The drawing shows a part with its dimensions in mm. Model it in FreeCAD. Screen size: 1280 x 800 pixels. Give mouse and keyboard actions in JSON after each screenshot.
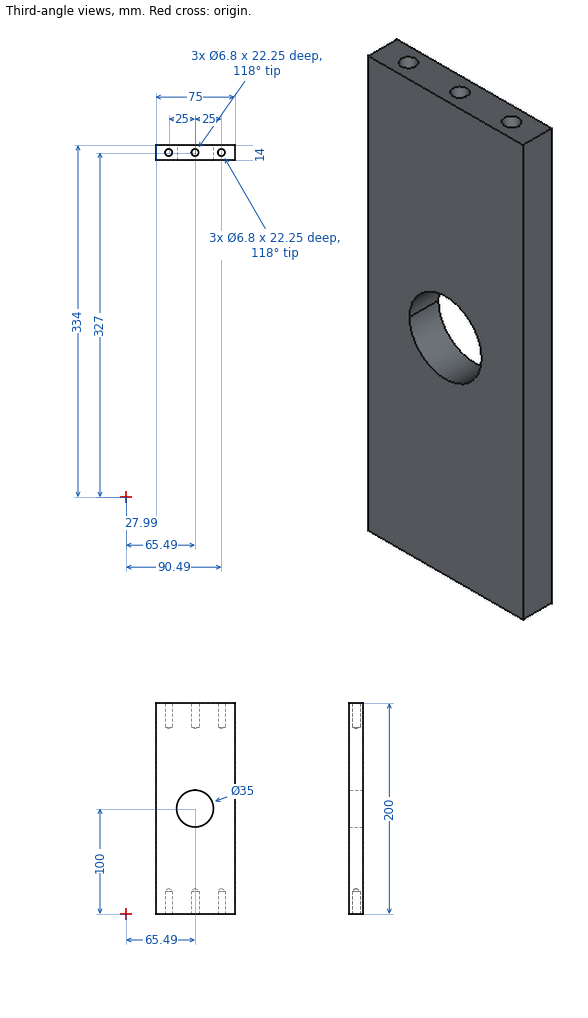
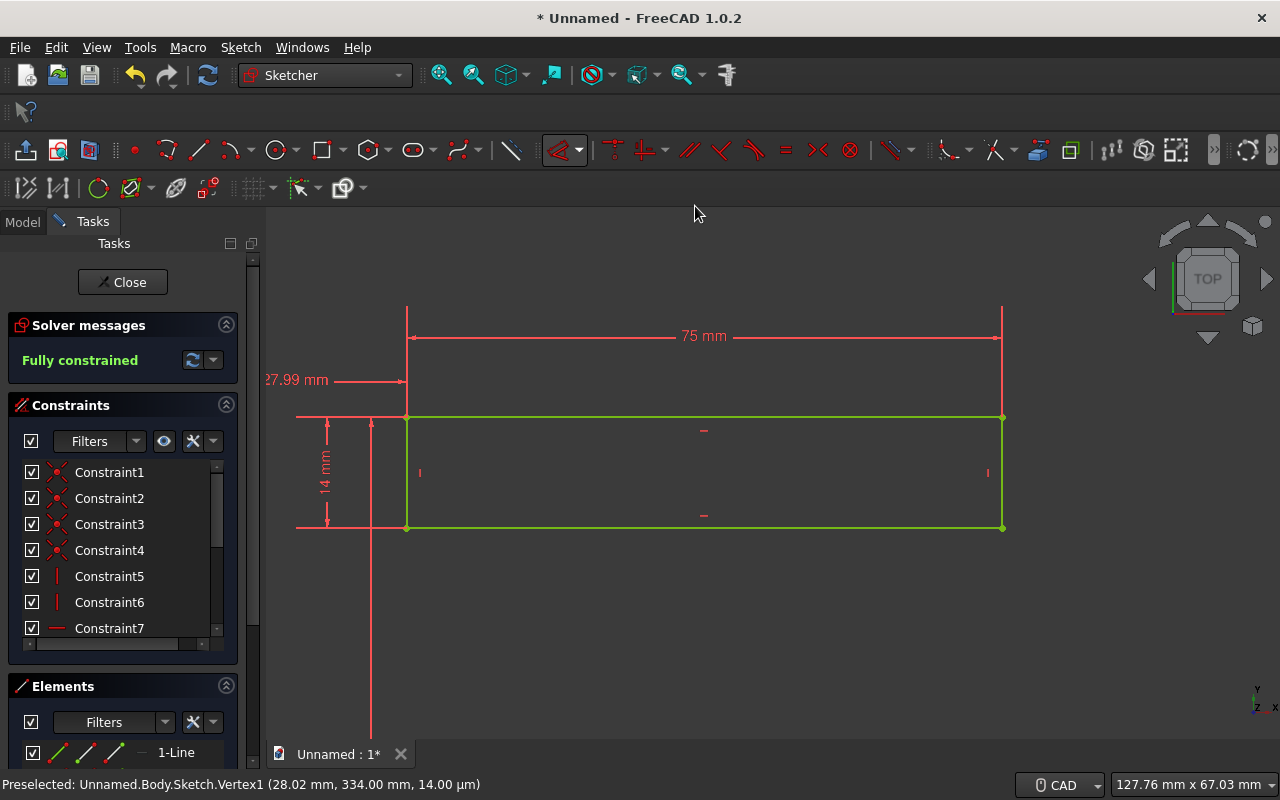
{"action": "left_click", "coordinate": [123, 282]}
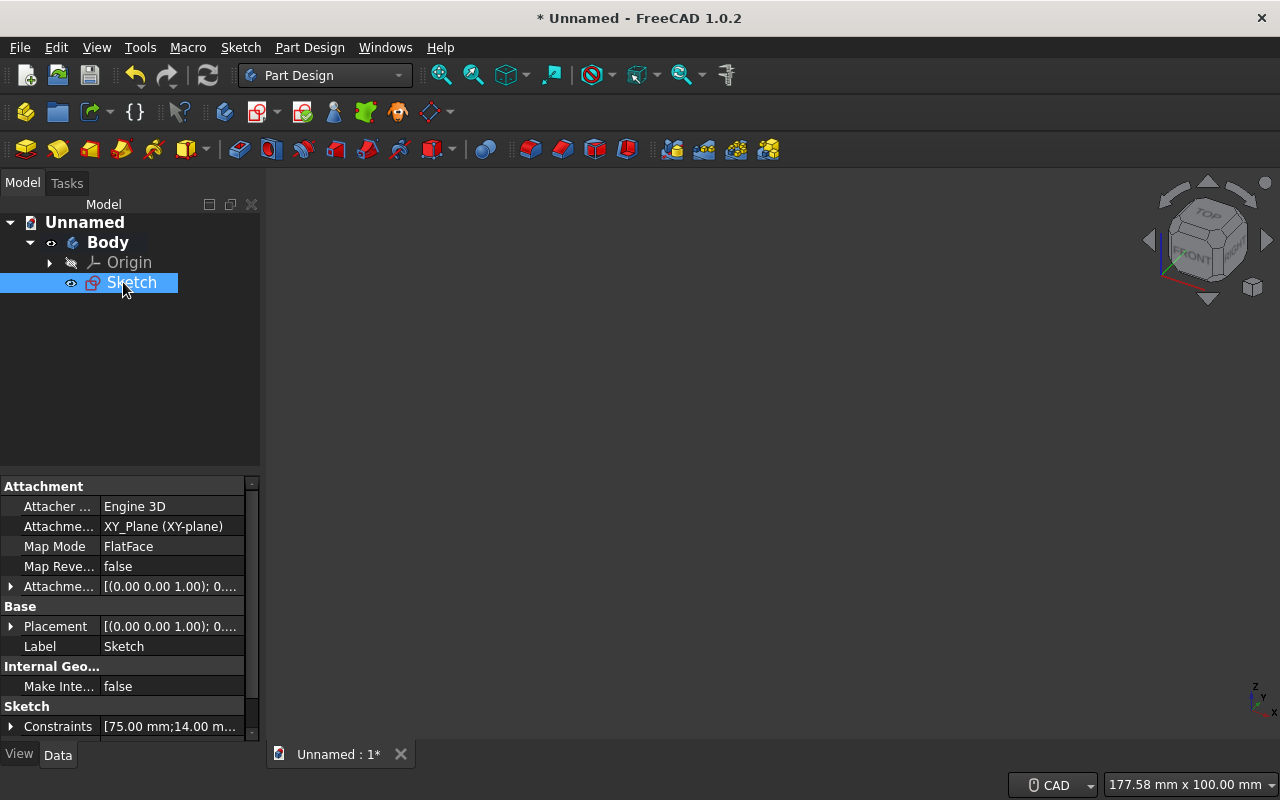
{"action": "left_click", "coordinate": [26, 150]}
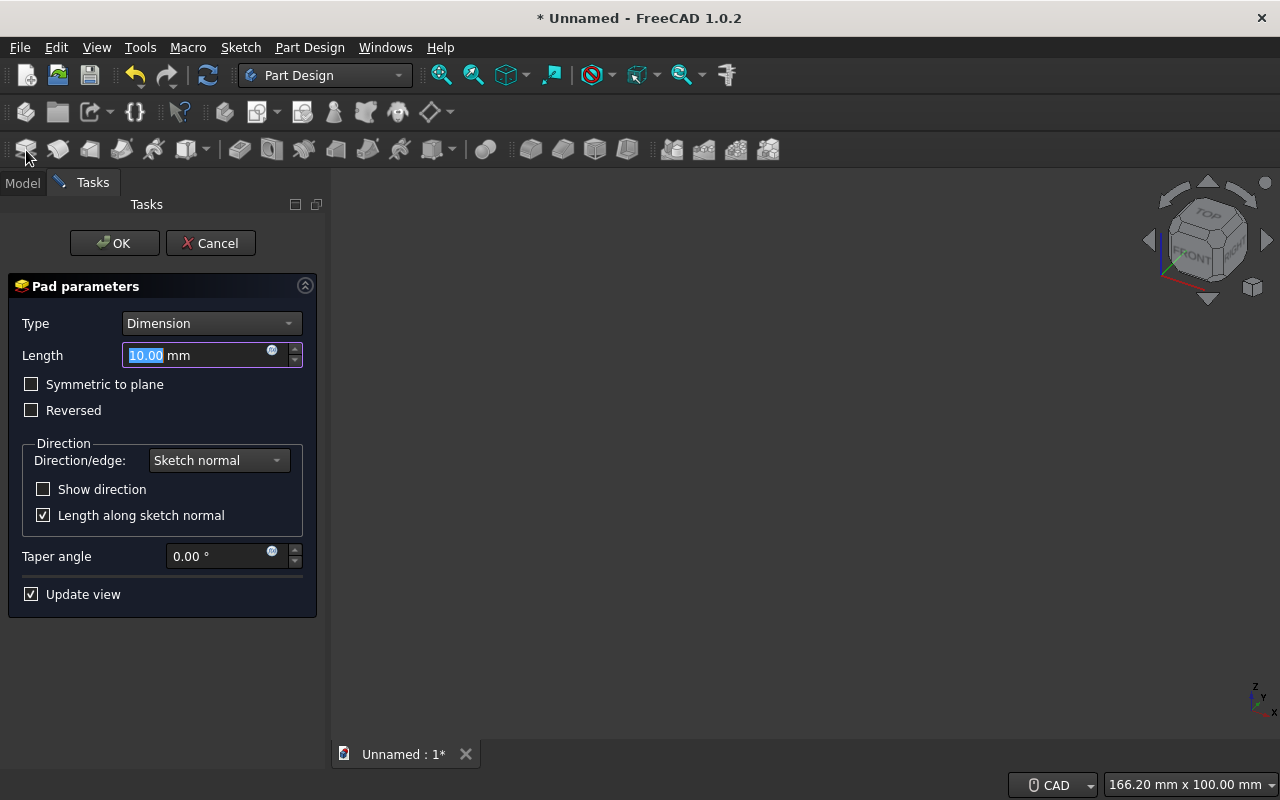
{"action": "type", "text": "200"}
{"action": "key", "text": "Tab"}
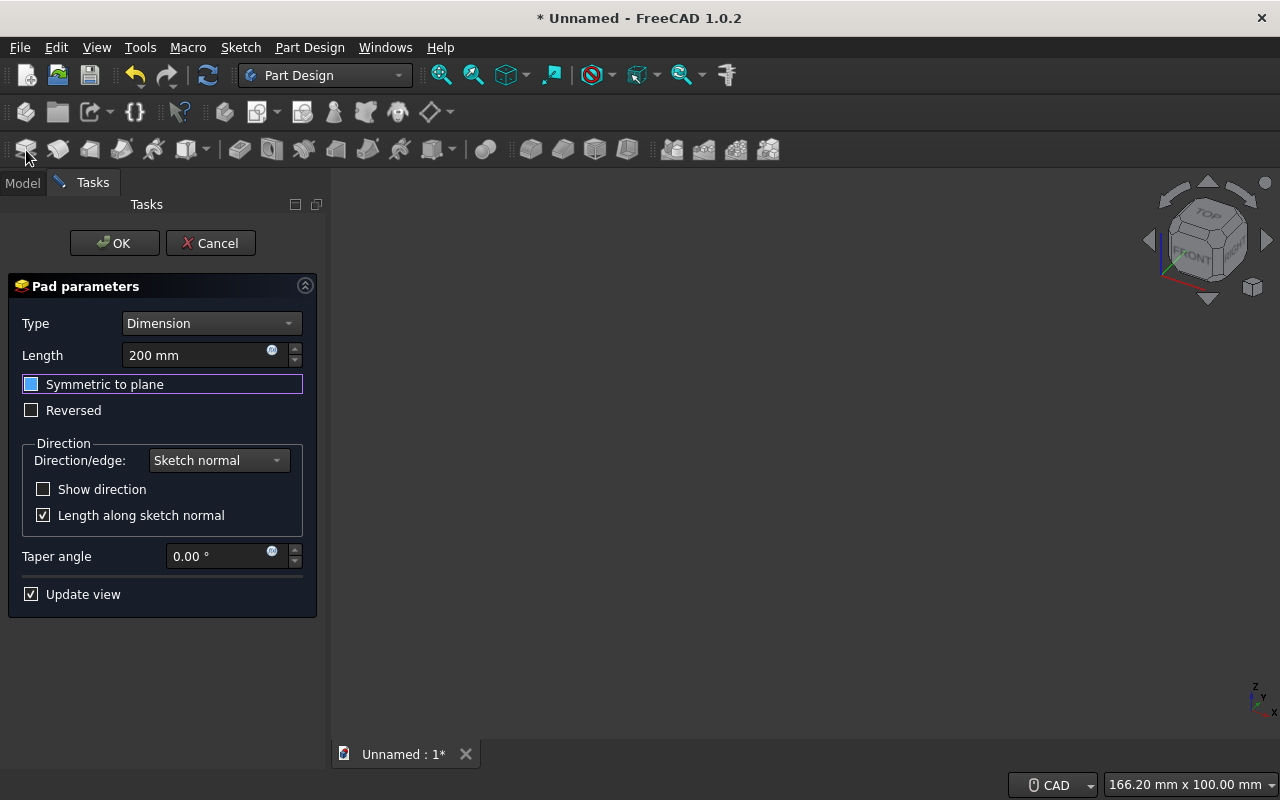
{"action": "left_click", "coordinate": [115, 243]}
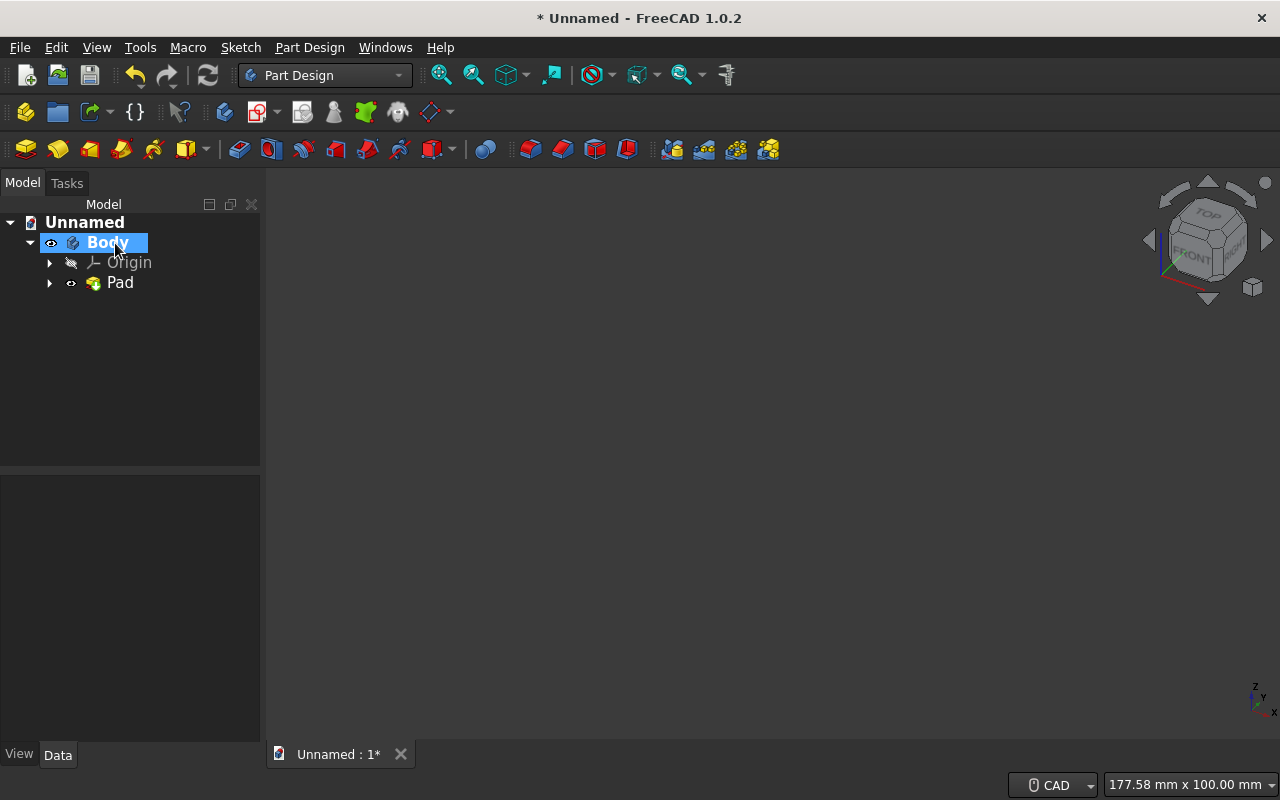
{"action": "left_click", "coordinate": [442, 76]}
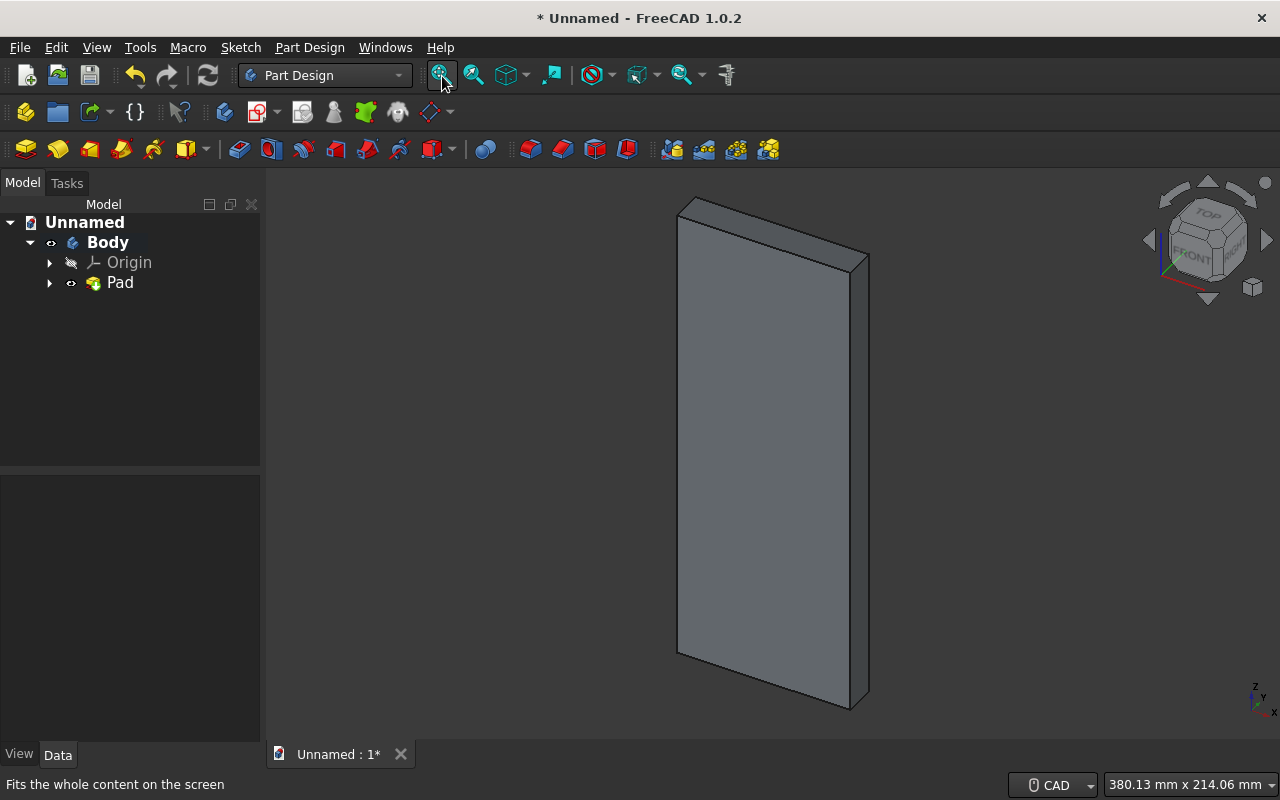
{"action": "key", "text": "4"}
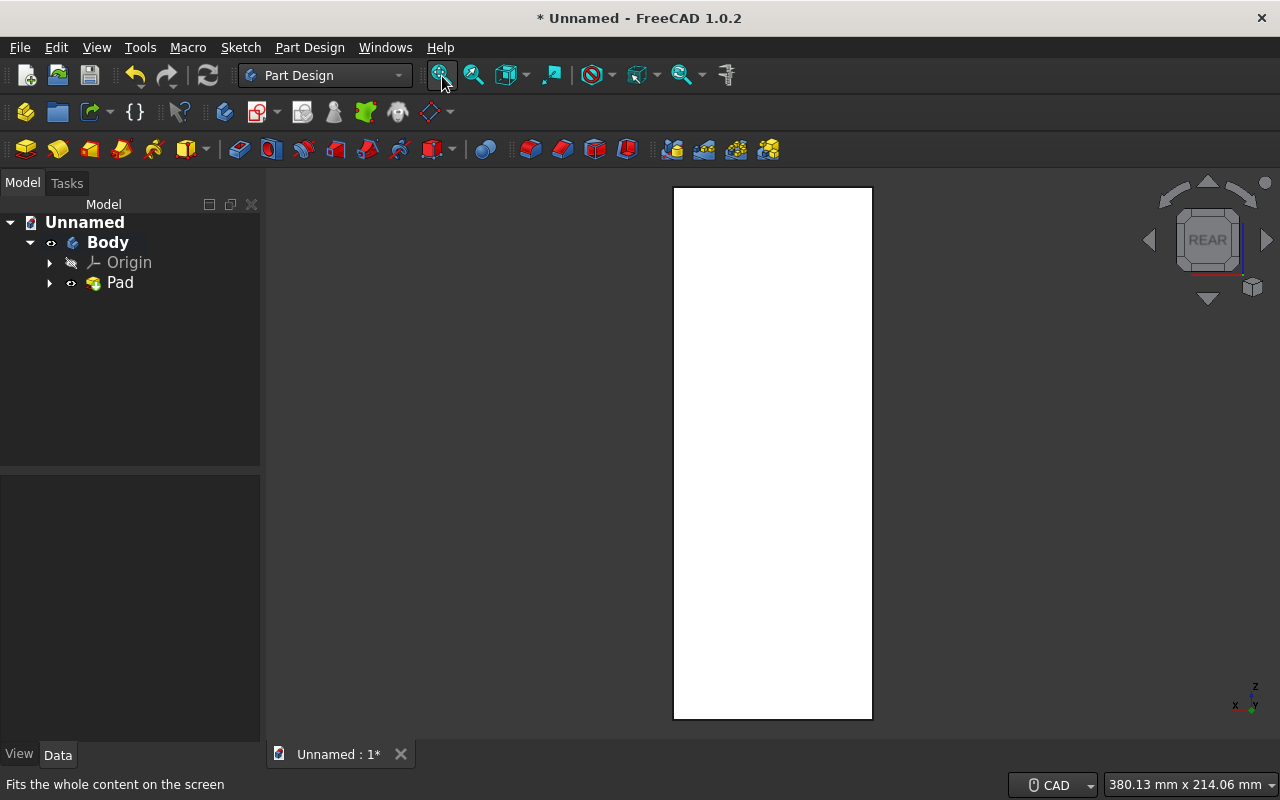
{"action": "left_click", "coordinate": [773, 300]}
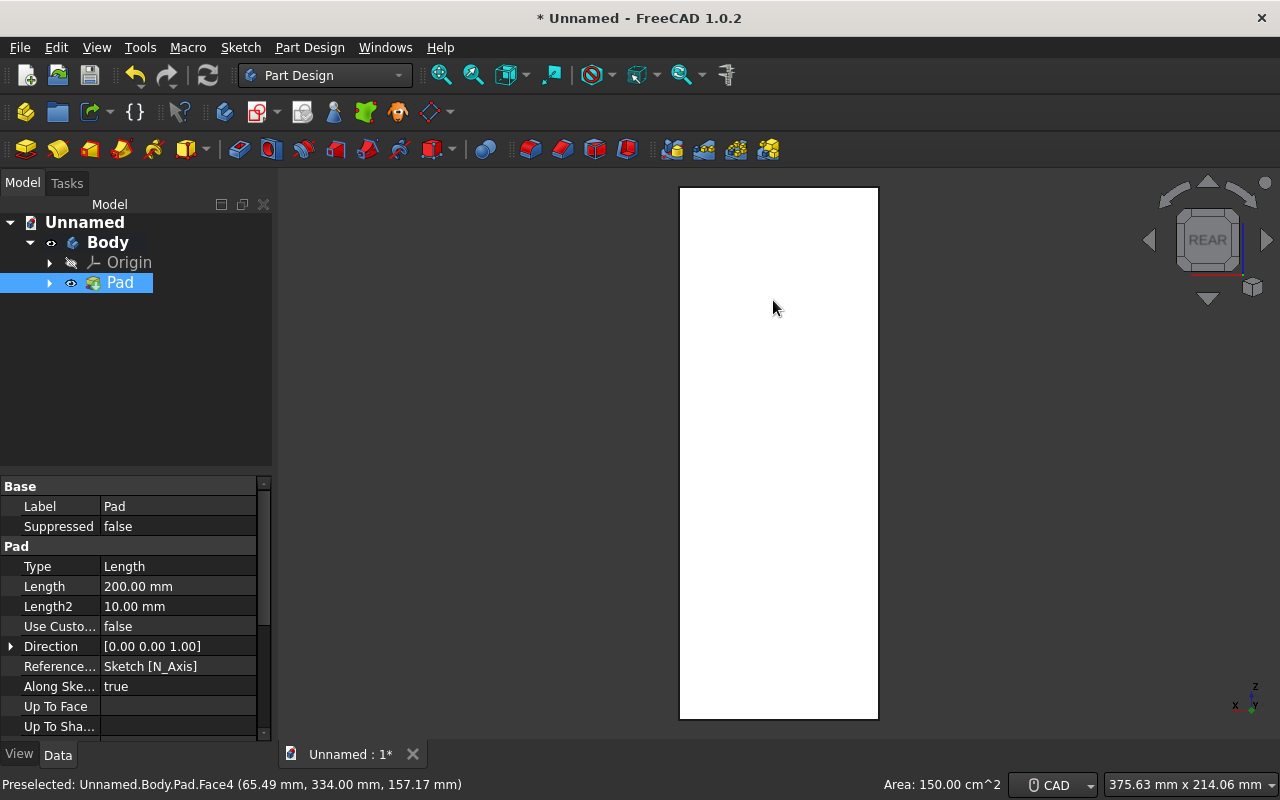
{"action": "left_click", "coordinate": [258, 112]}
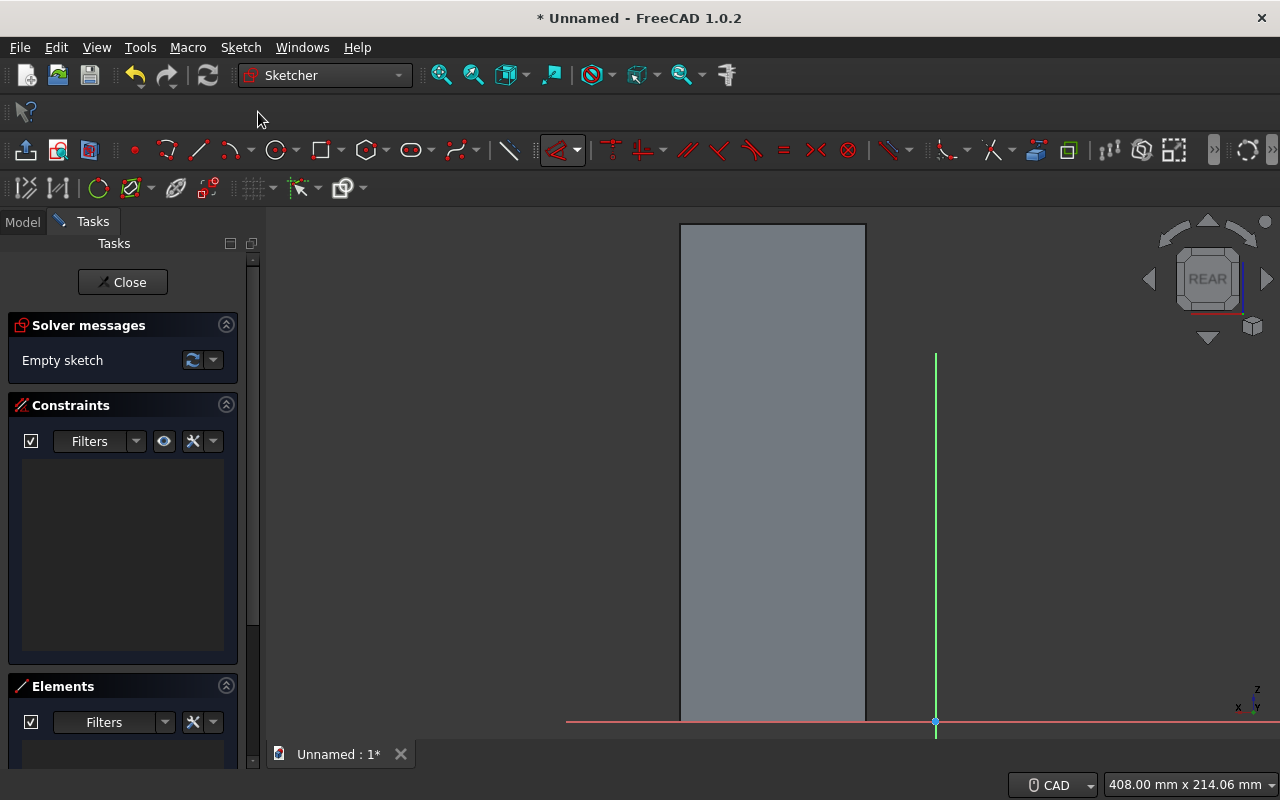
{"action": "scroll", "coordinate": [795, 473], "scroll_direction": "up", "scroll_amount": 7}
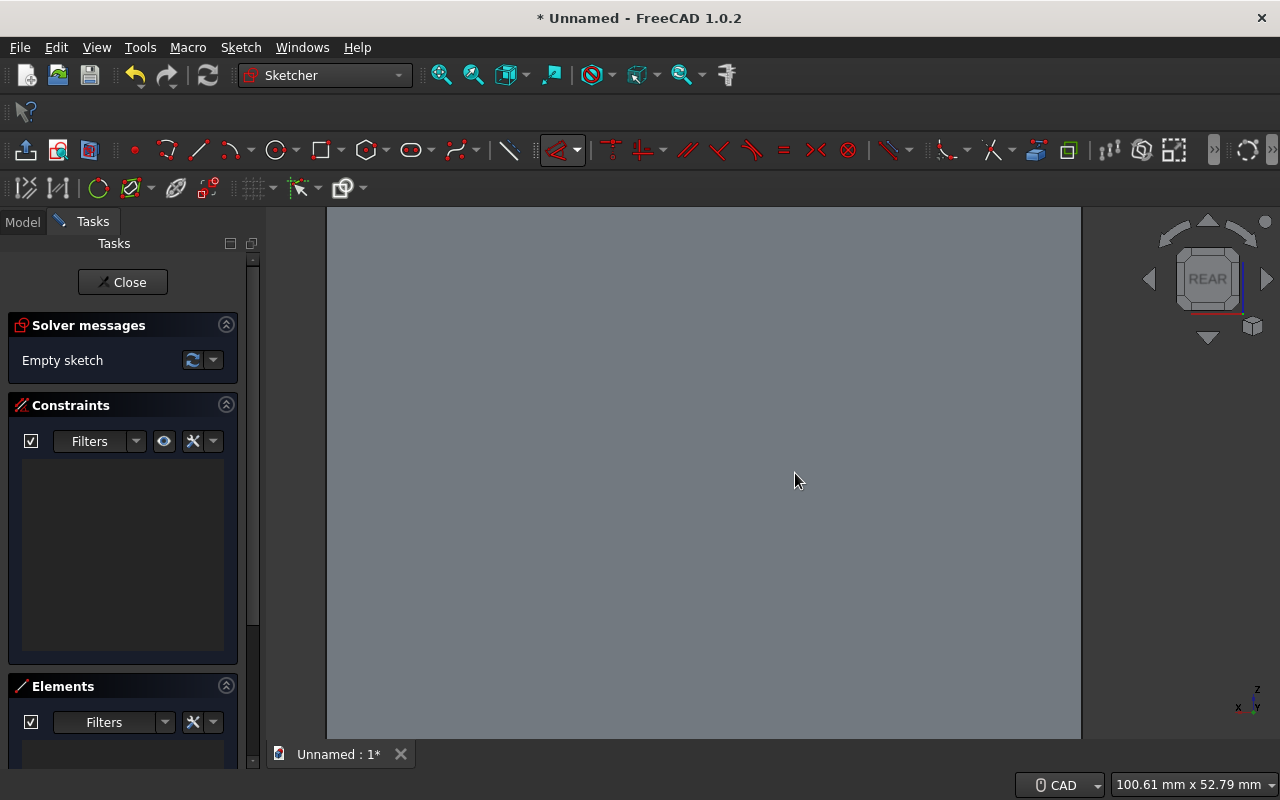
{"action": "left_click", "coordinate": [276, 150]}